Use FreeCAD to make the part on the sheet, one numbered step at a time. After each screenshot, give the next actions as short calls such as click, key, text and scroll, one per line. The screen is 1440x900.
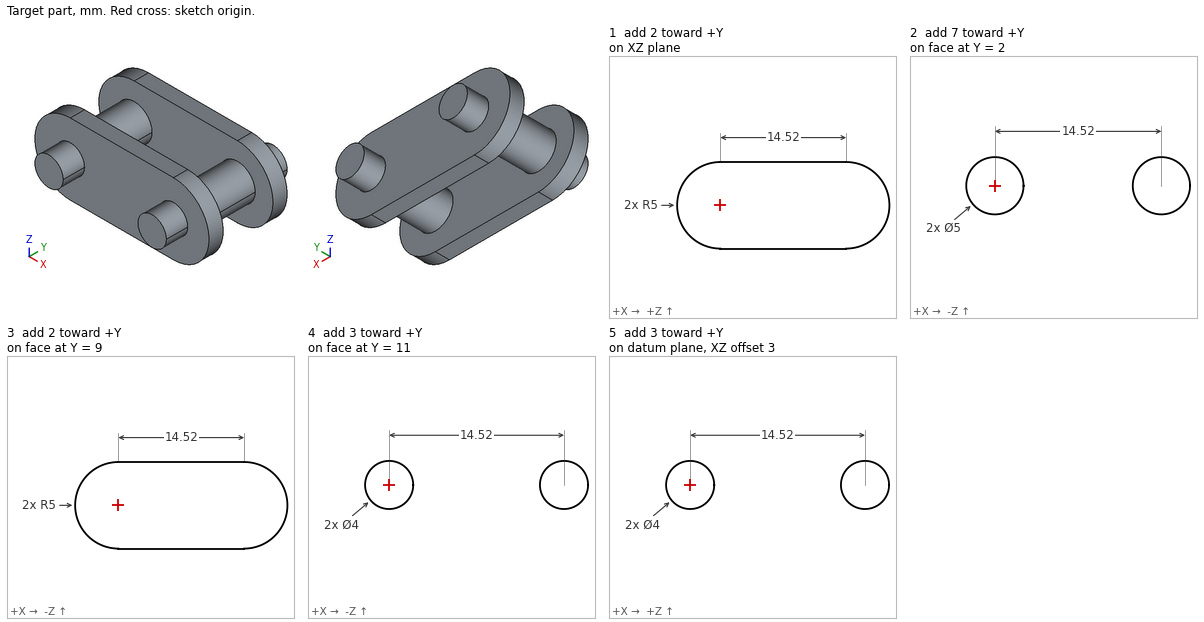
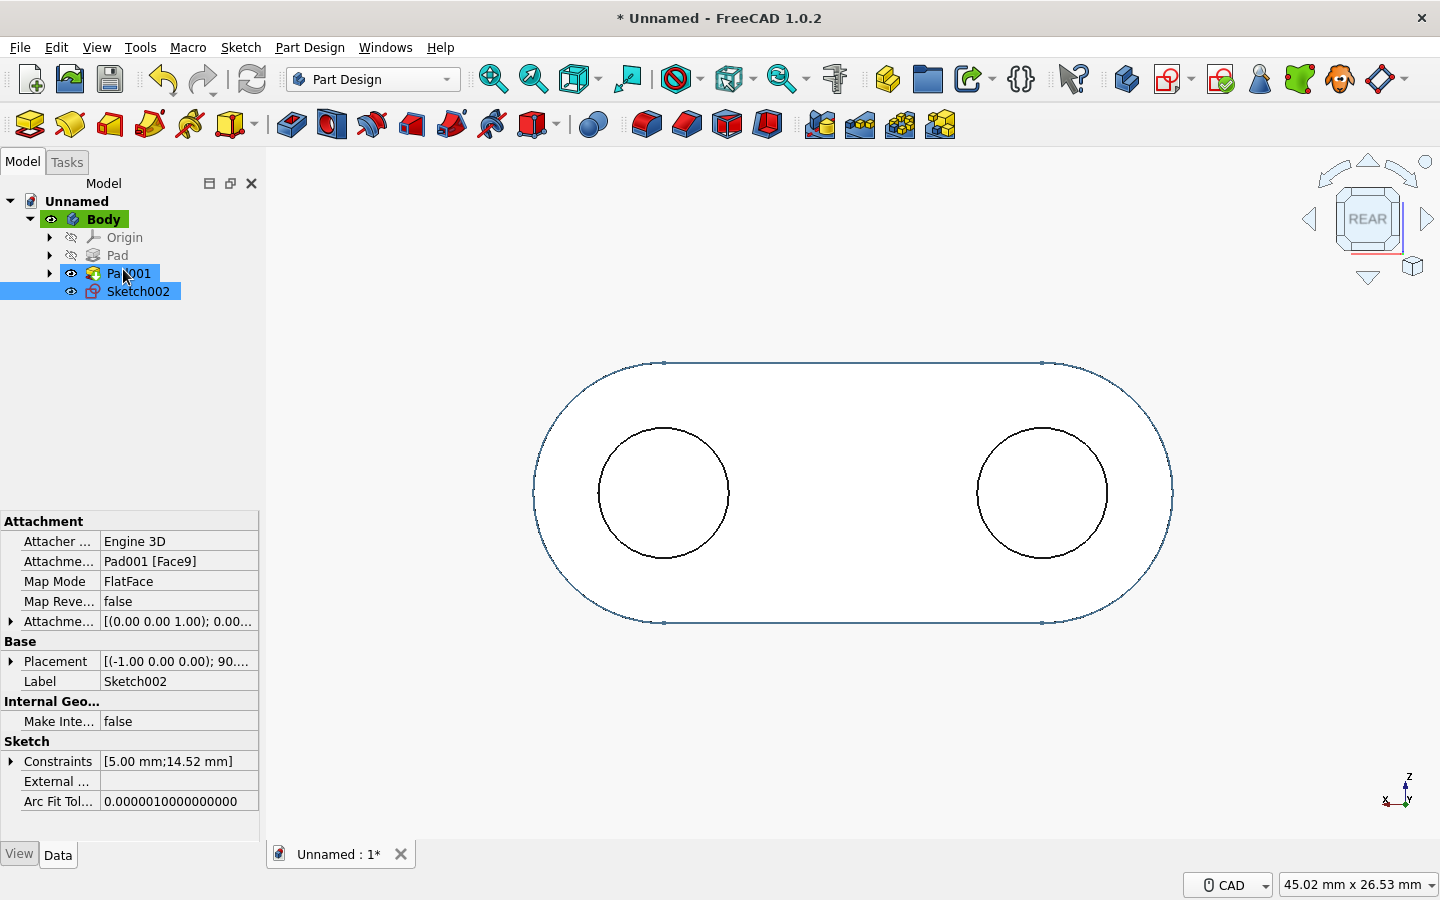
click(30, 124)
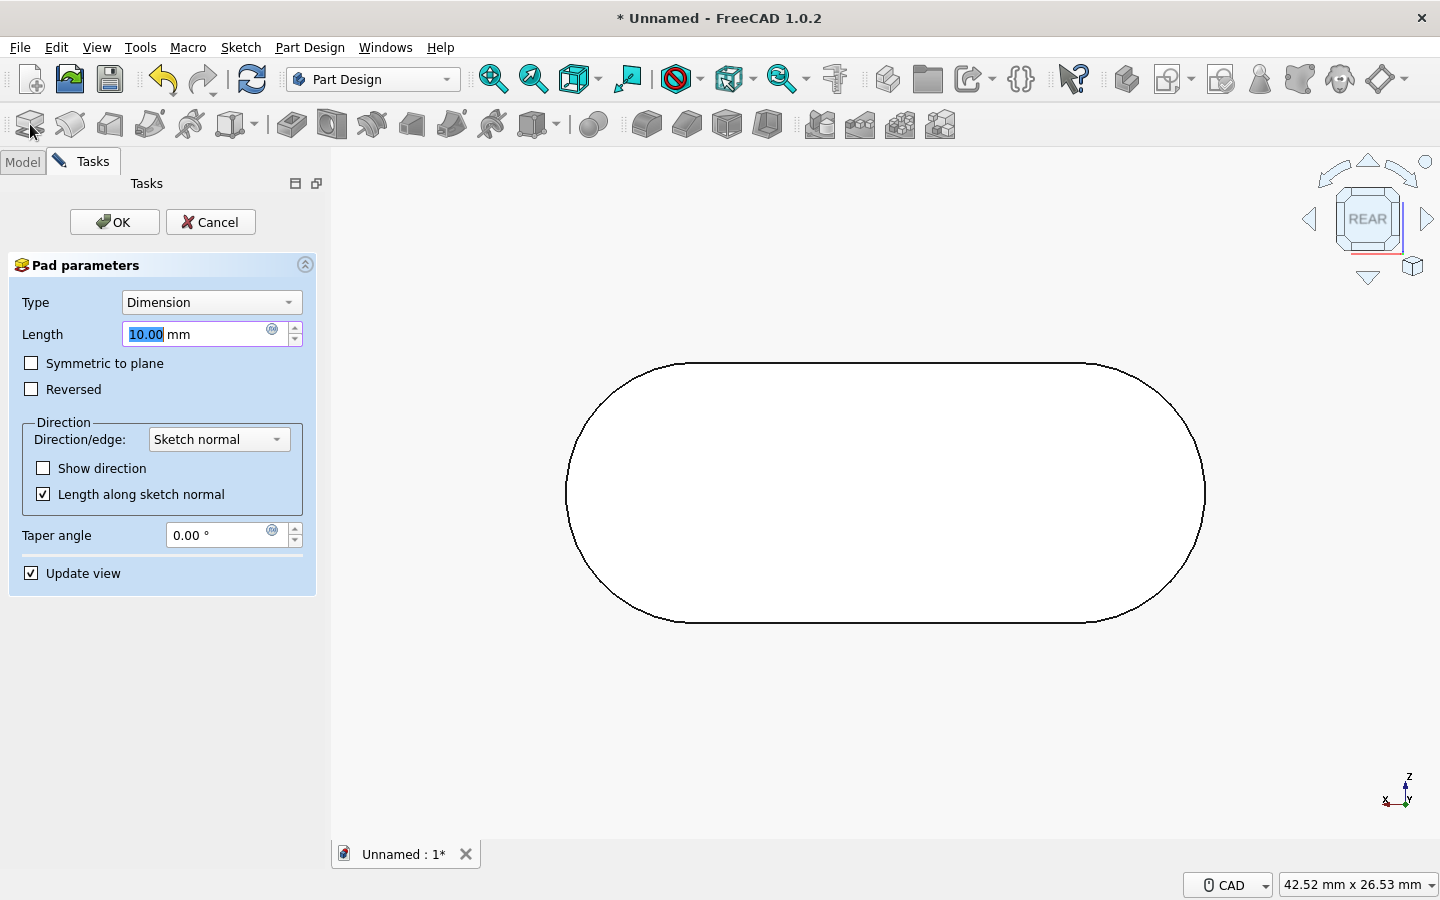
text(2)
key(Tab)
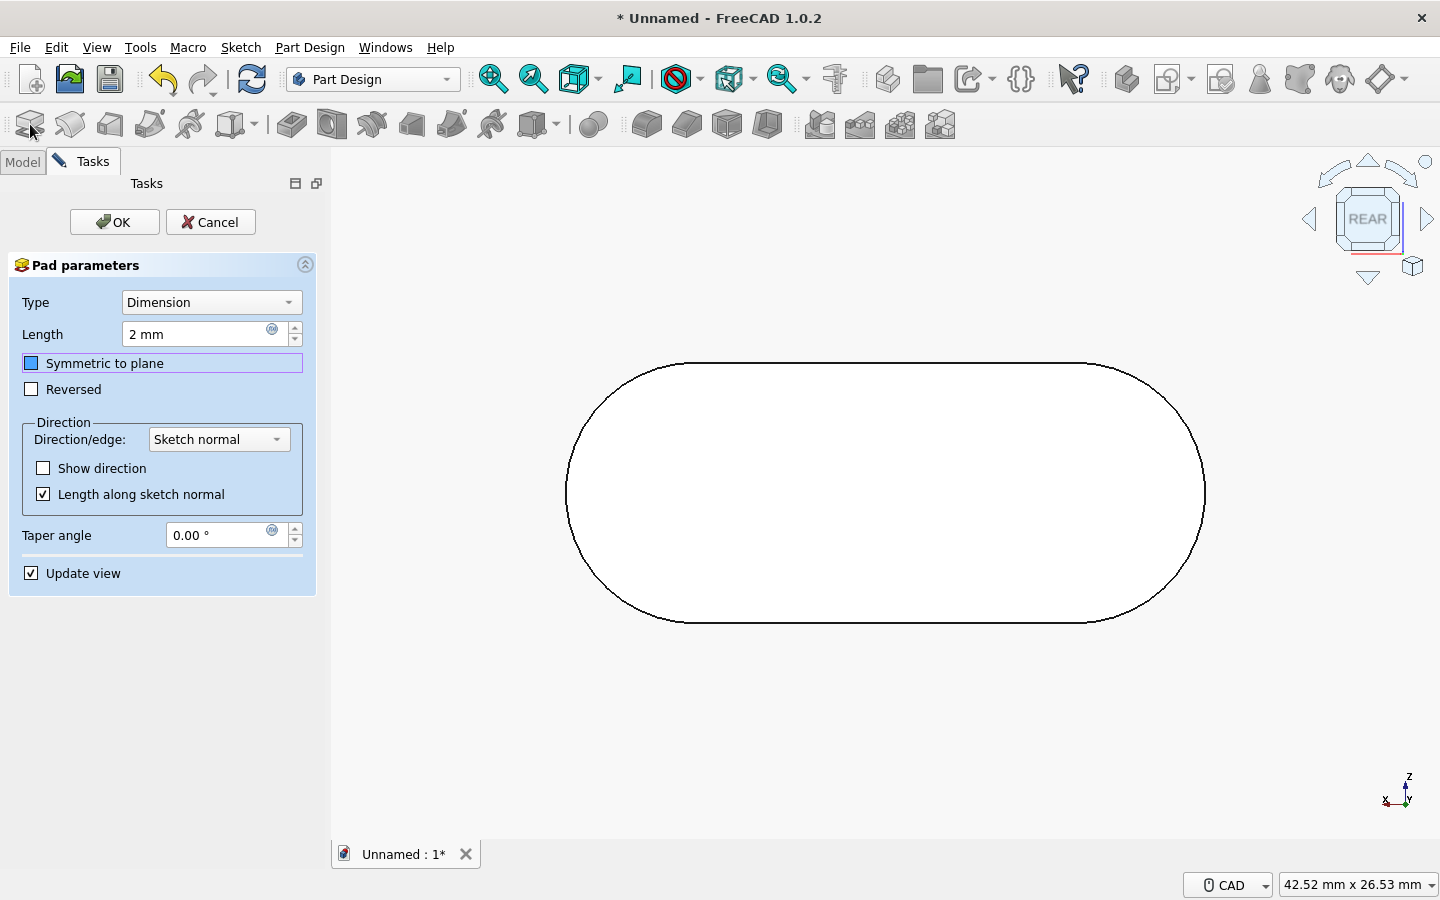
click(115, 222)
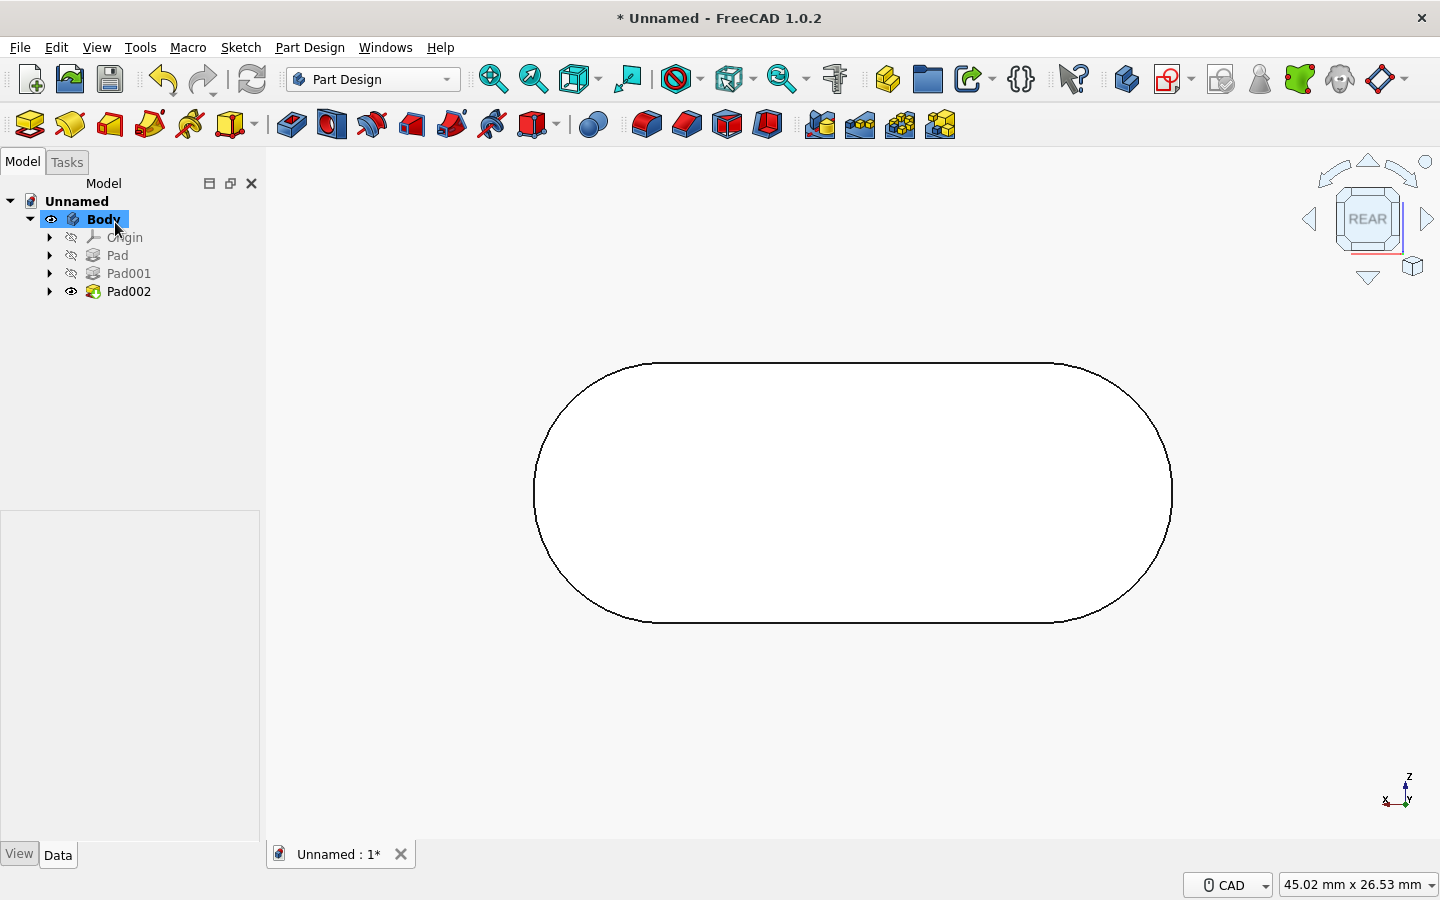
click(670, 492)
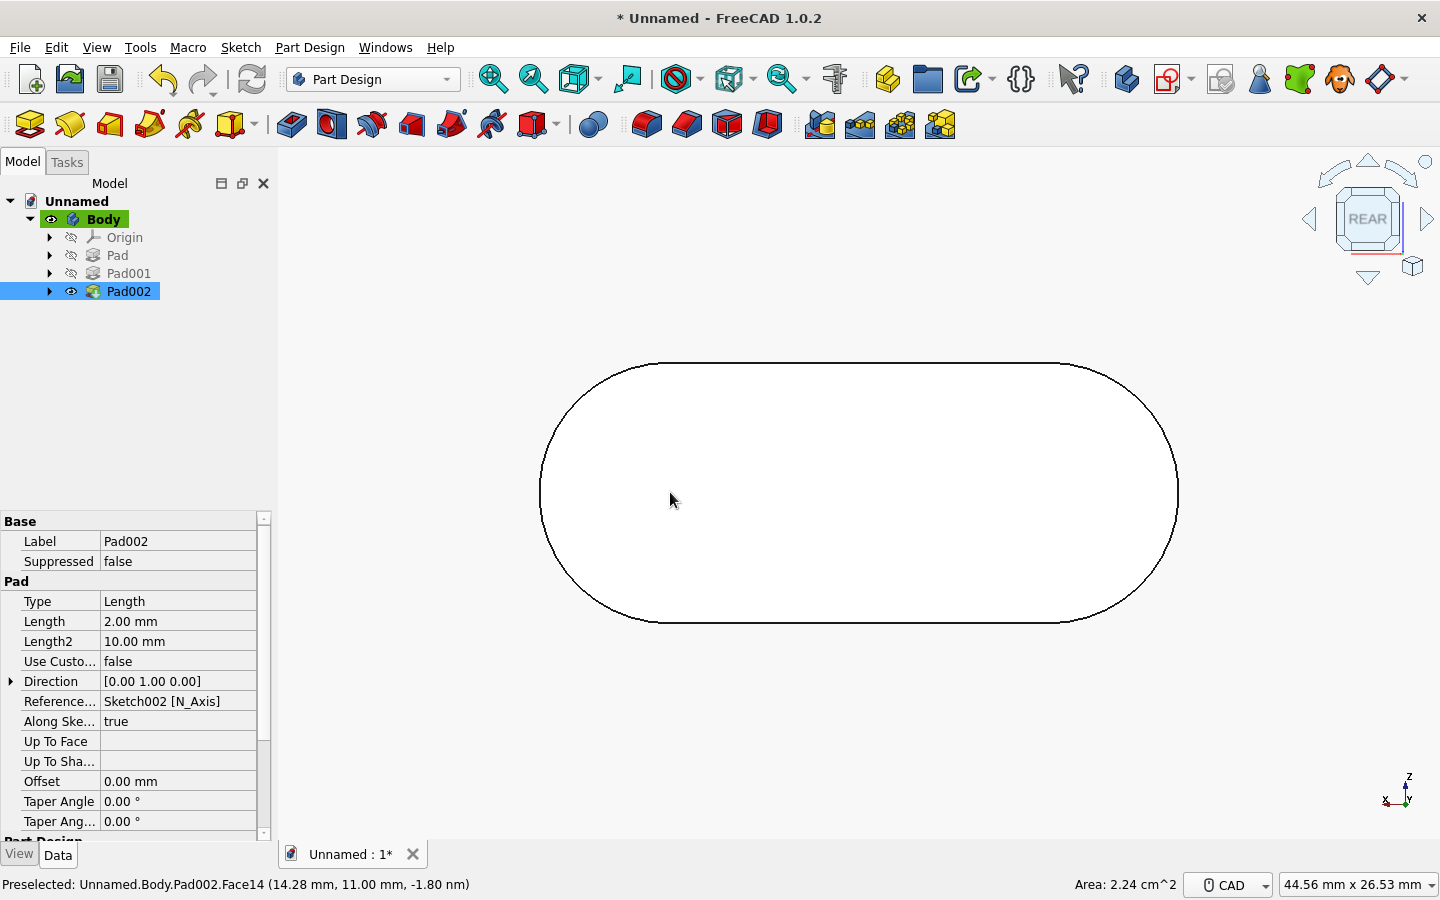
click(1168, 80)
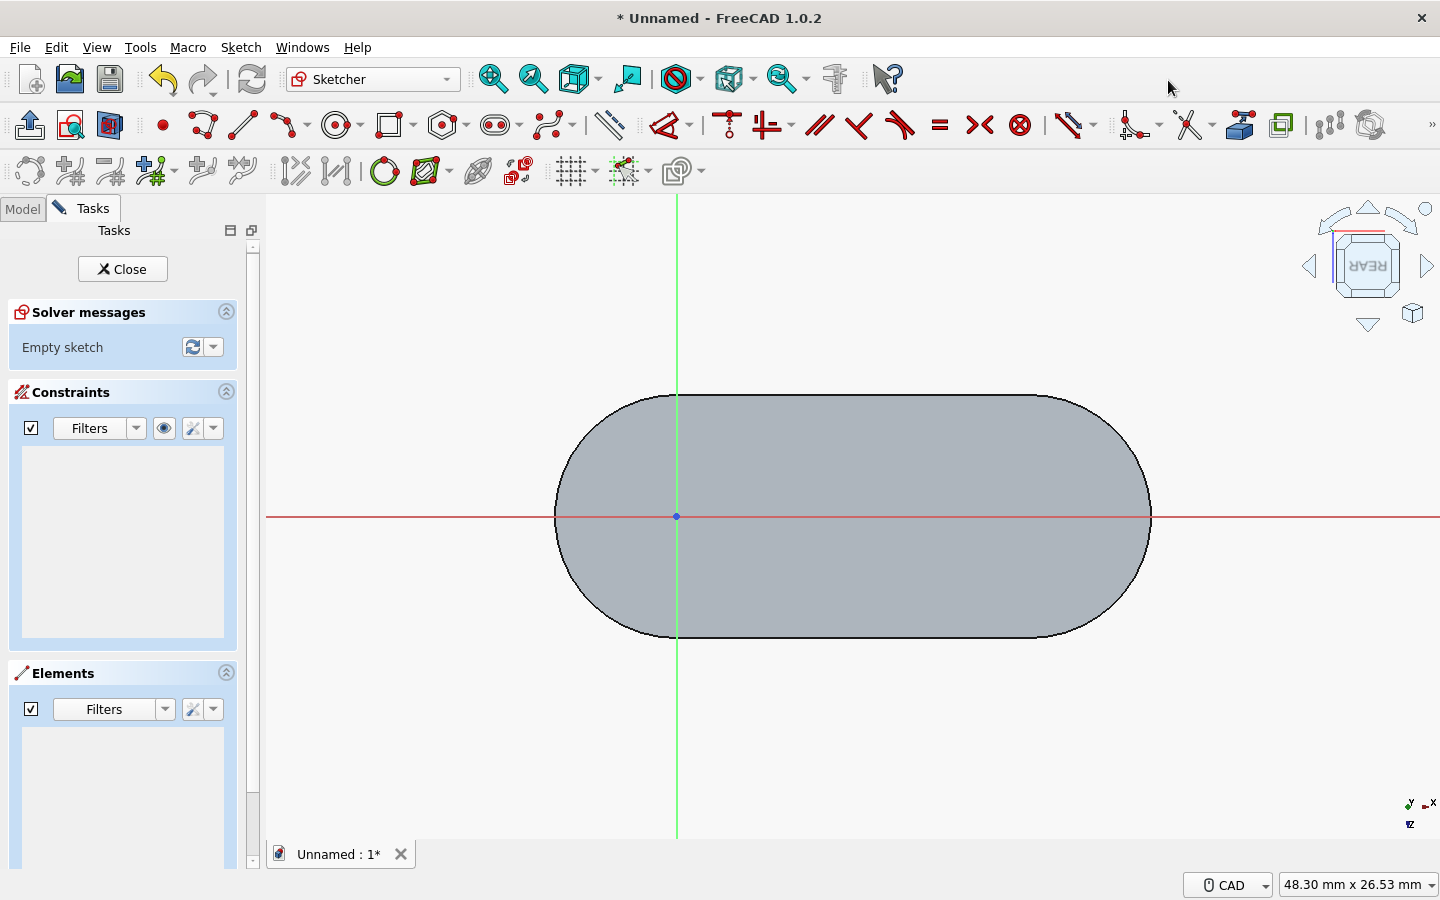
scroll(992, 516, up, 2)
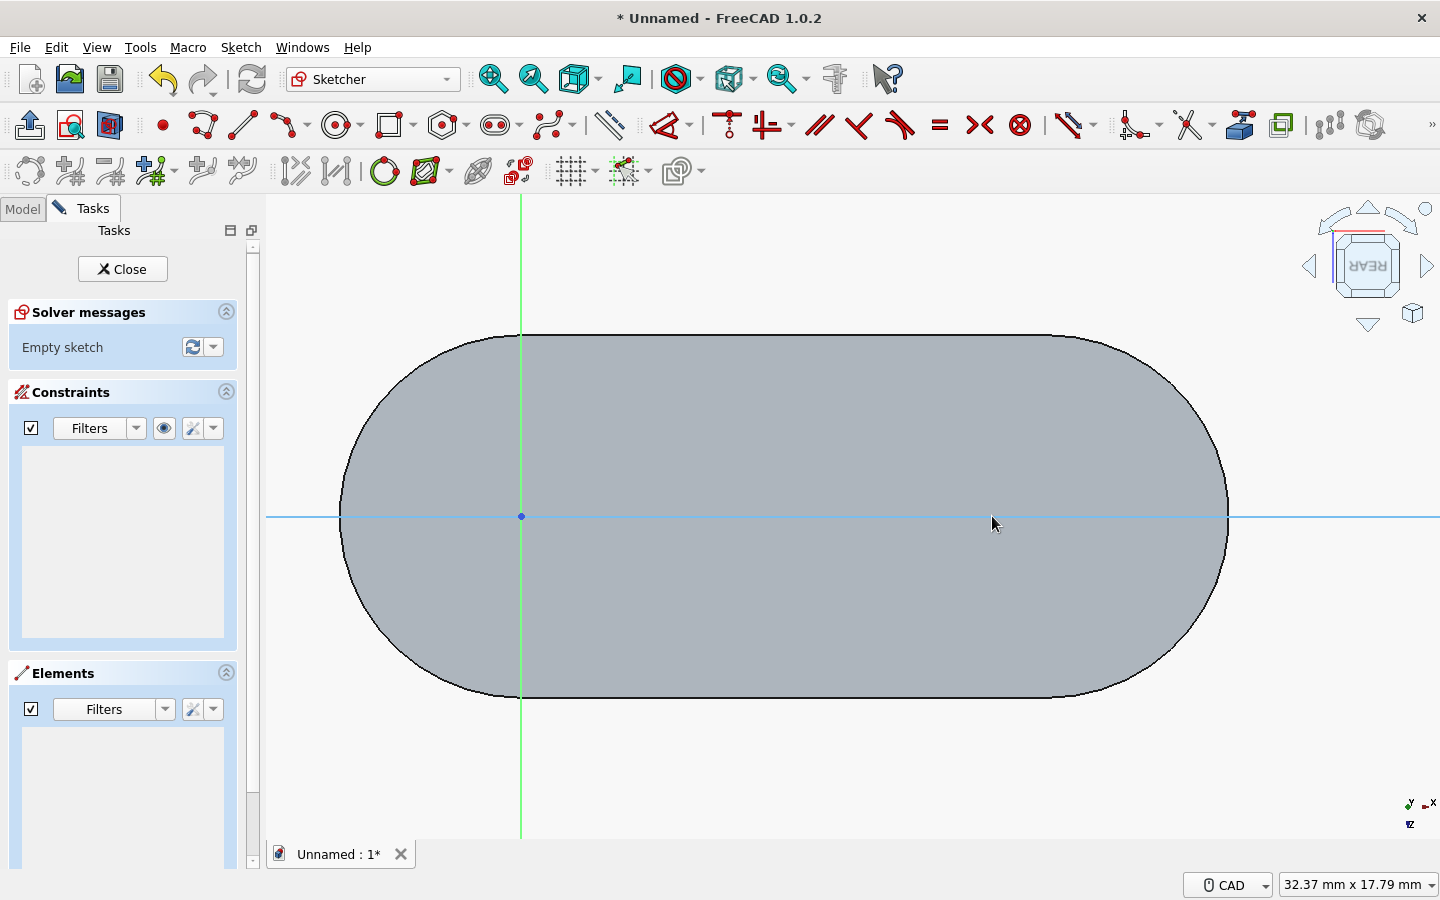
key(g)
key(c)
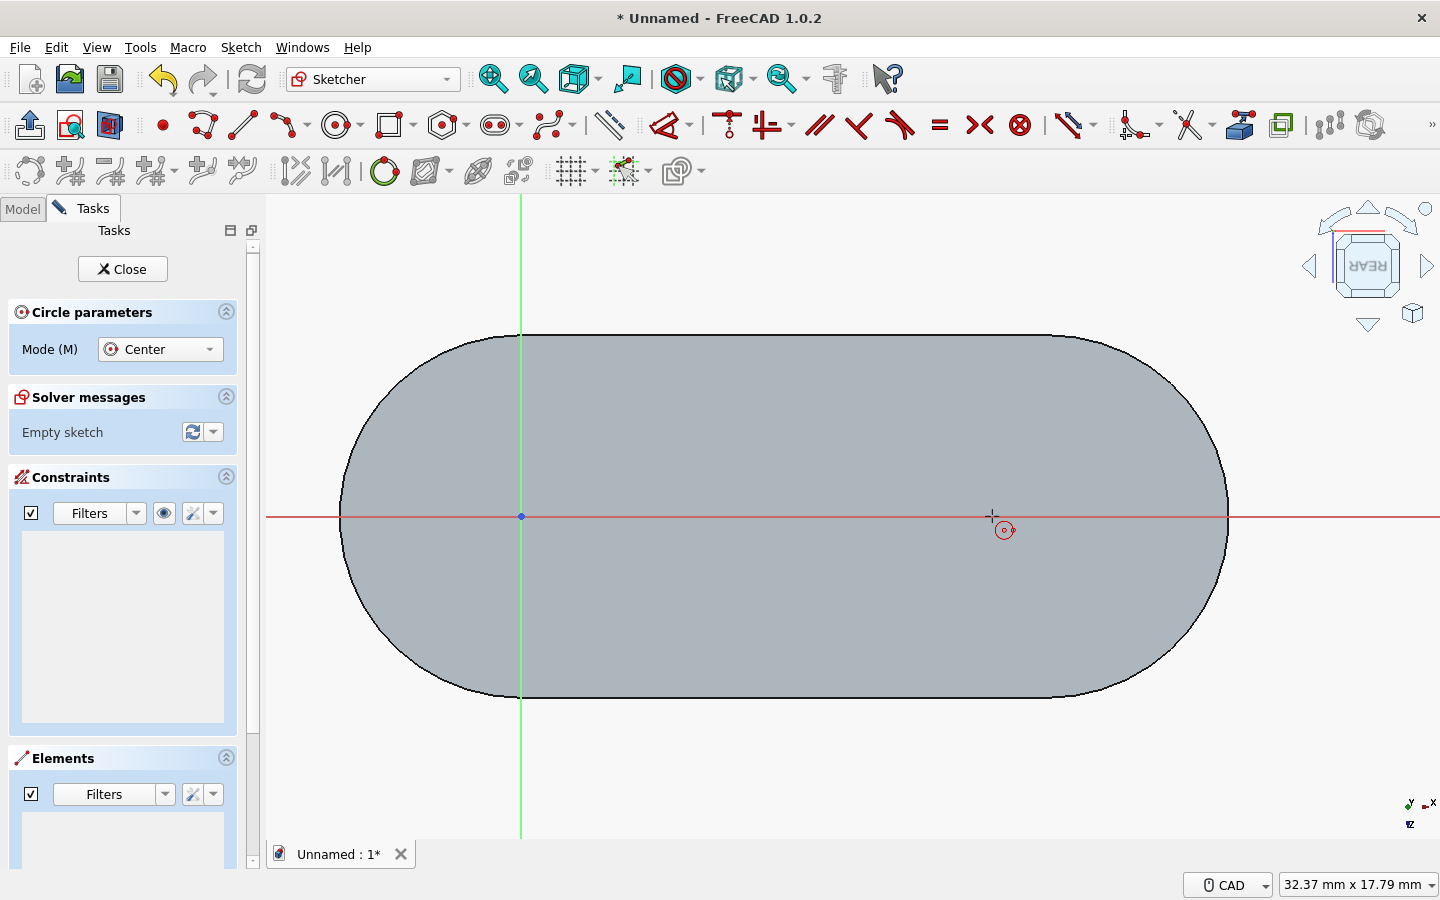
click(521, 516)
move(572, 465)